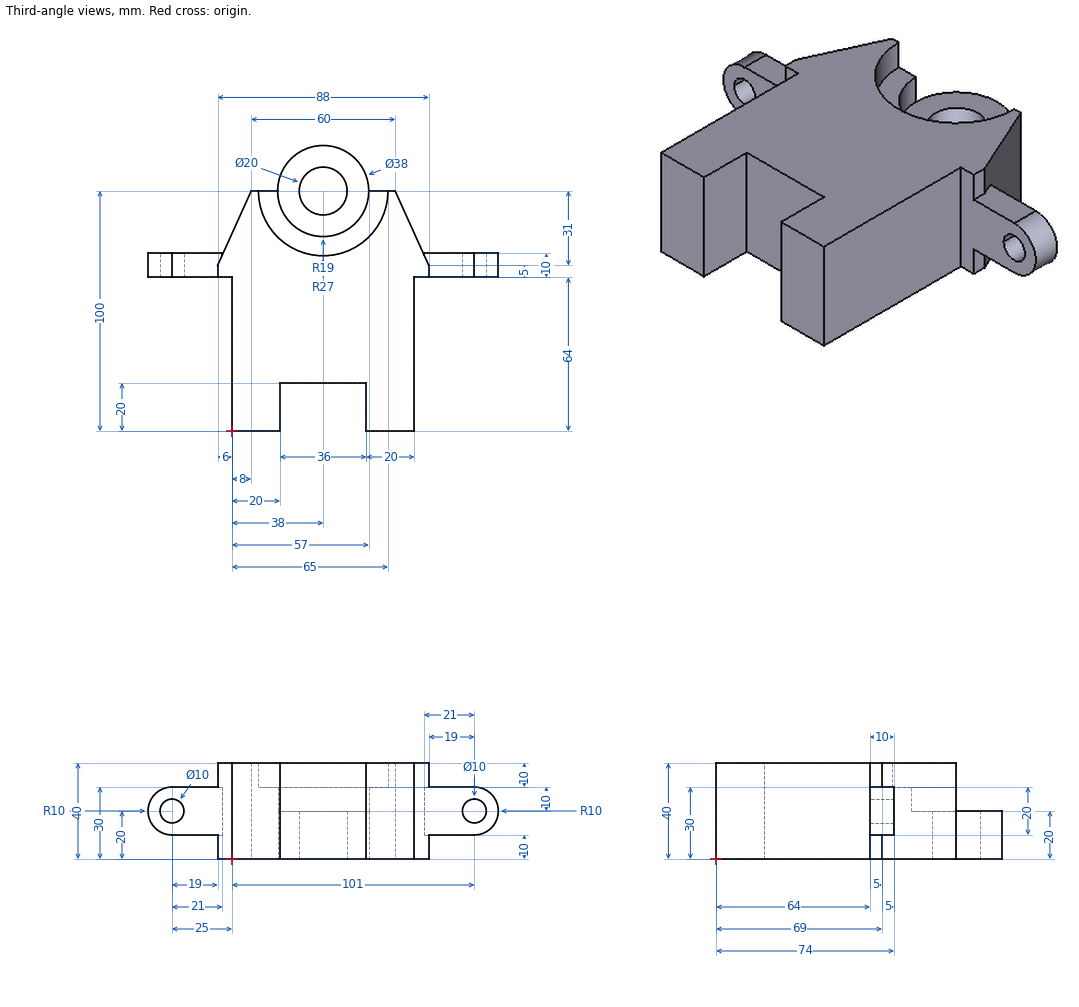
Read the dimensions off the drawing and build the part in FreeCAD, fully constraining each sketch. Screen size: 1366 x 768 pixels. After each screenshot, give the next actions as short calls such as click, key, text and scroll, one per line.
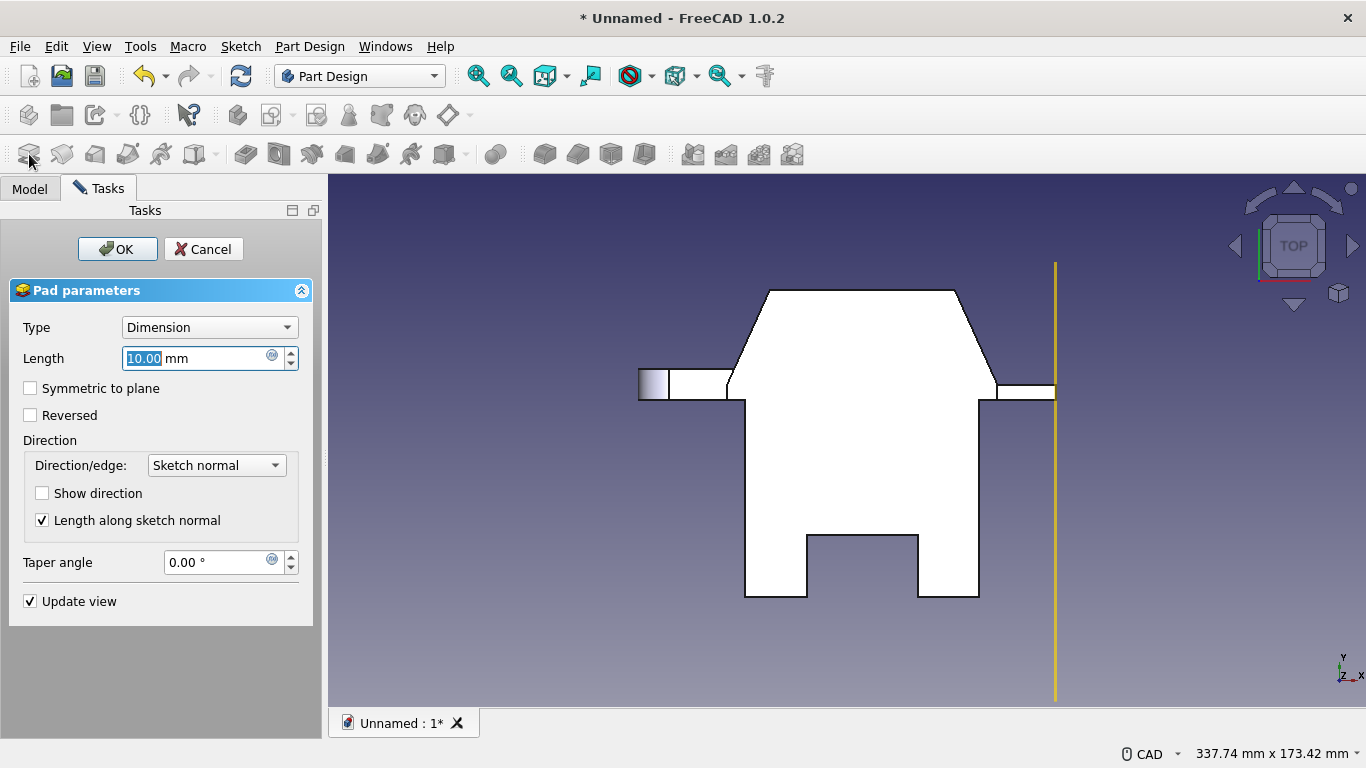
text(21)
key(Tab)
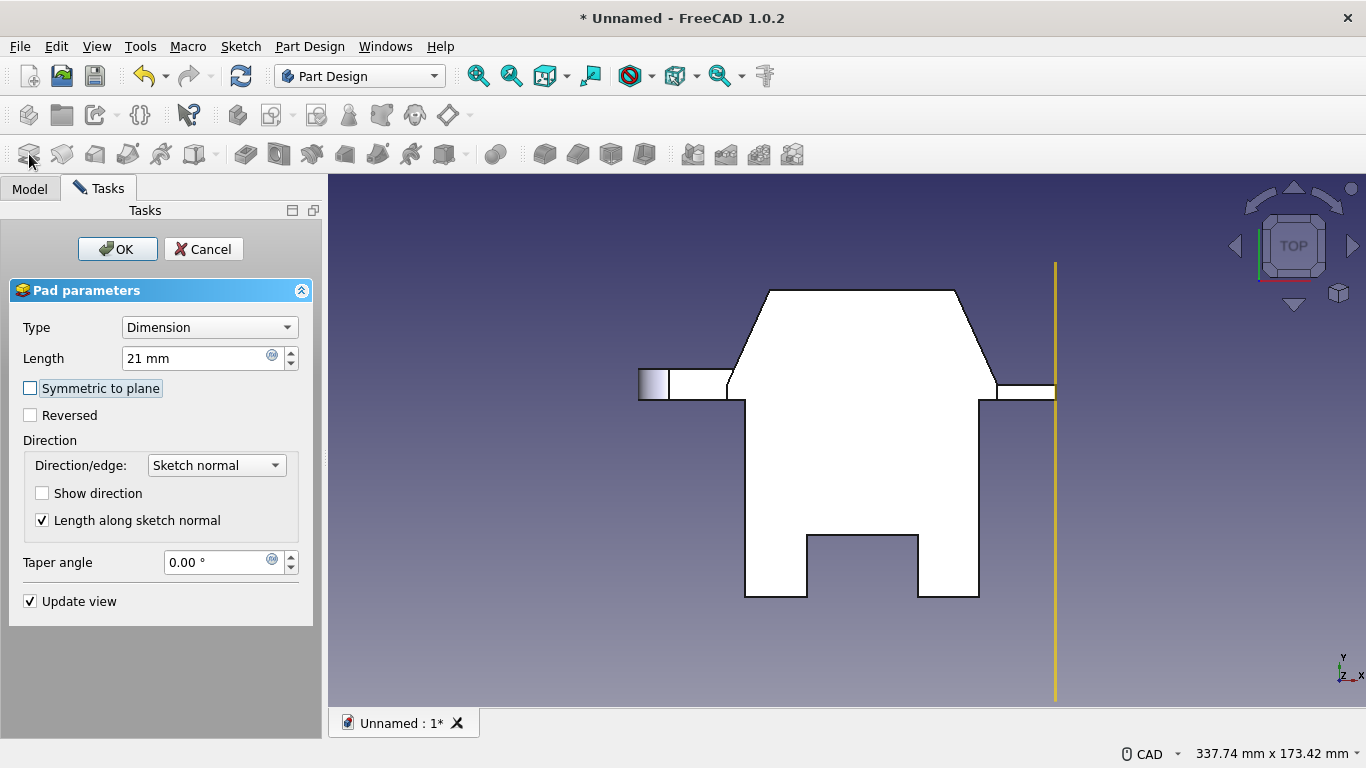
click(31, 415)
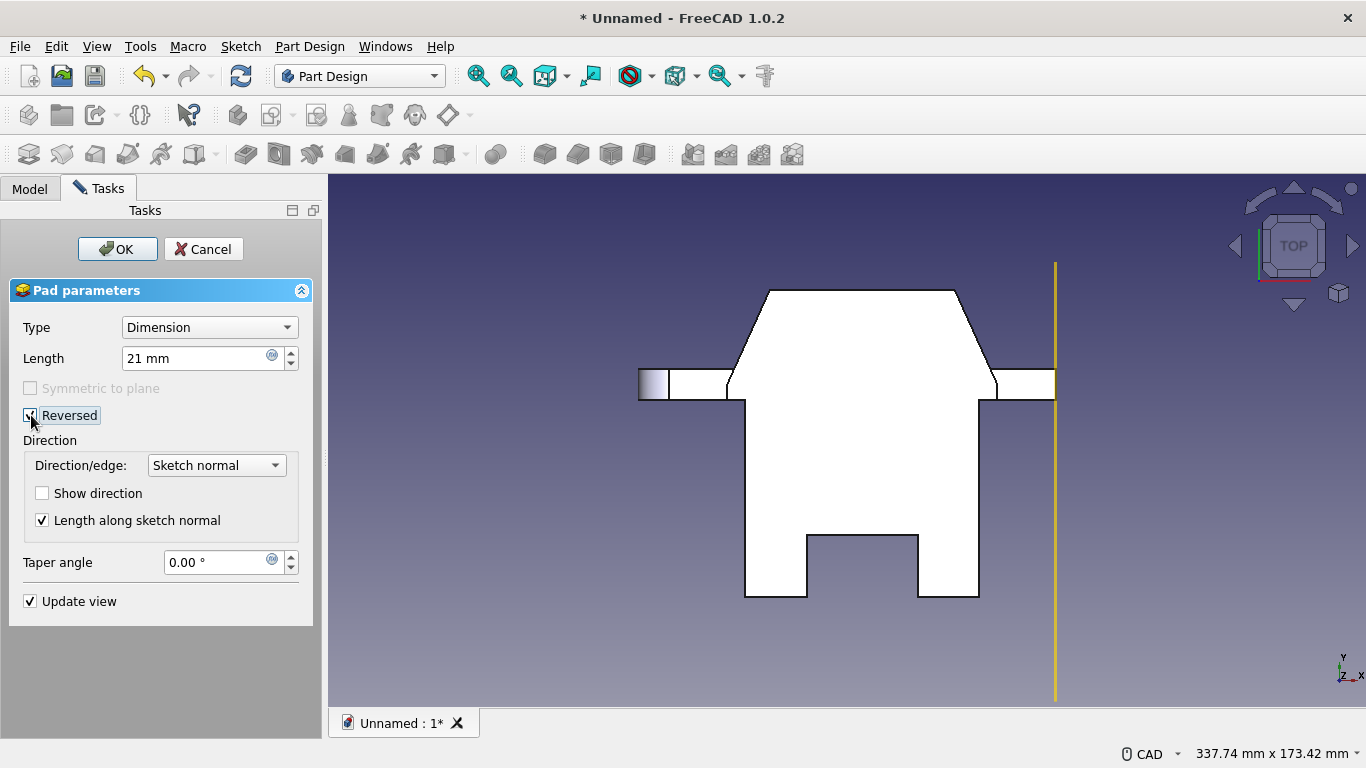
click(118, 249)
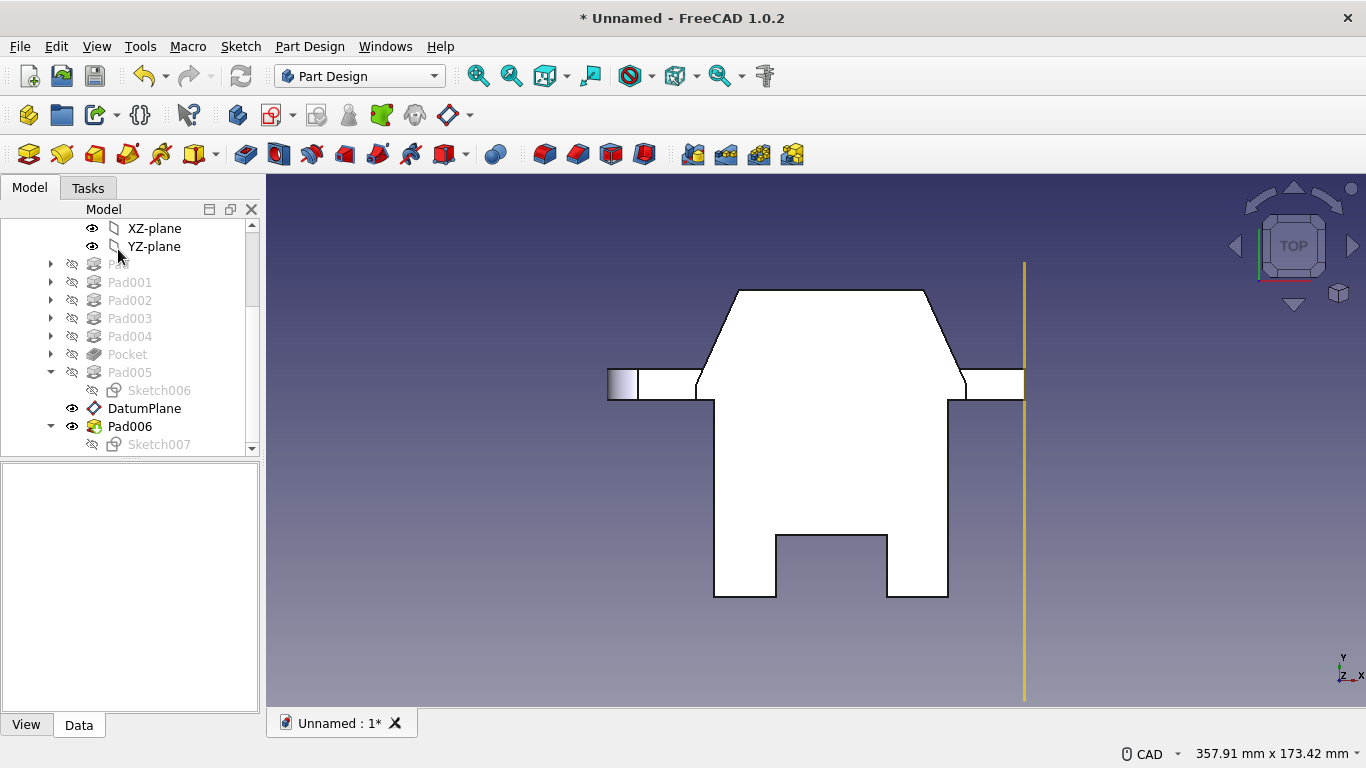
click(117, 408)
key(space)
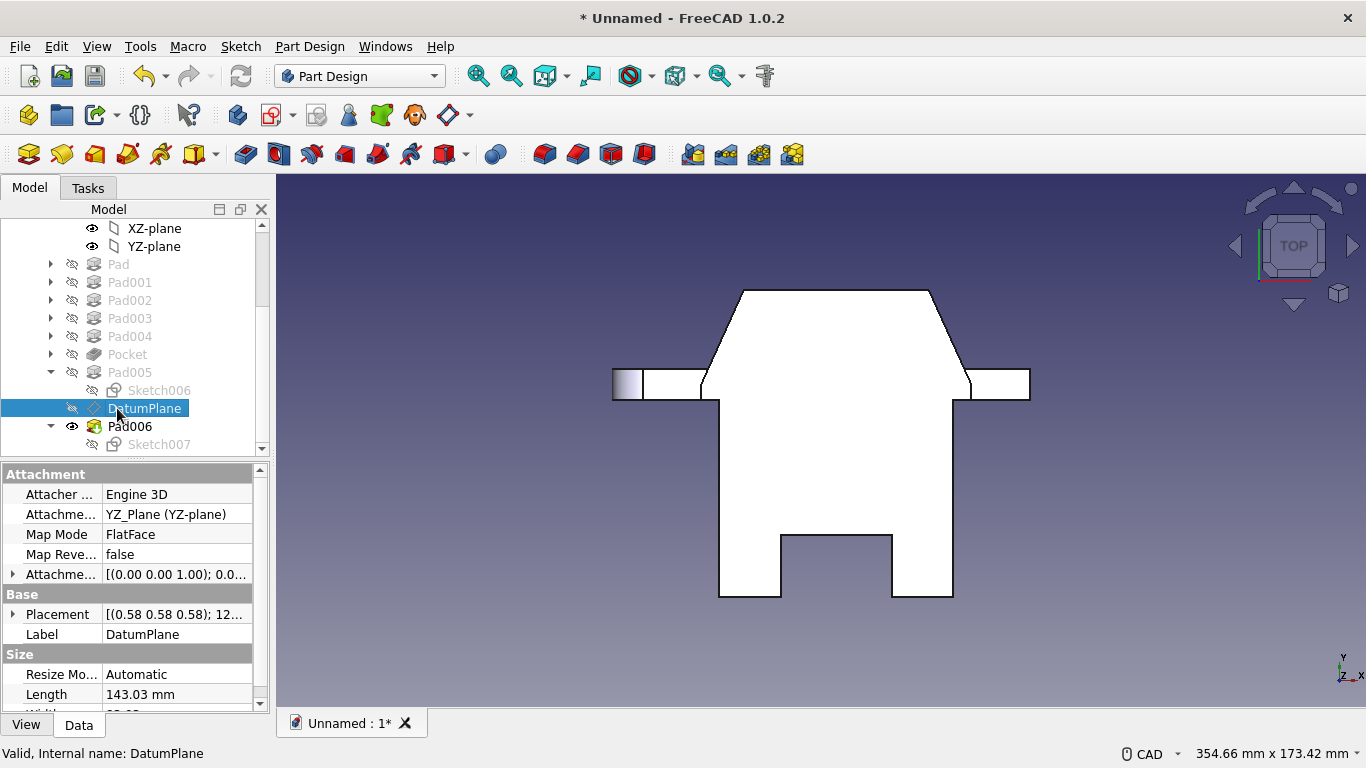
key(4)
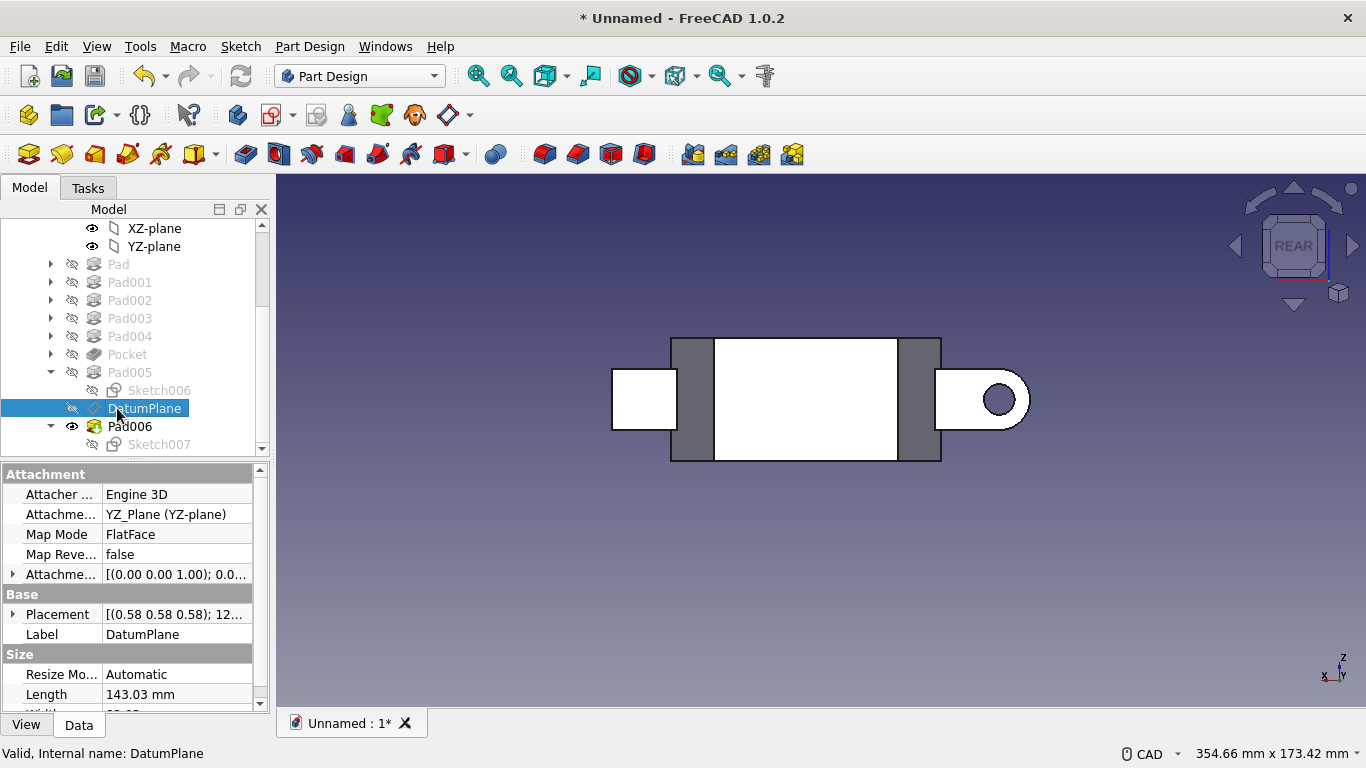
click(479, 76)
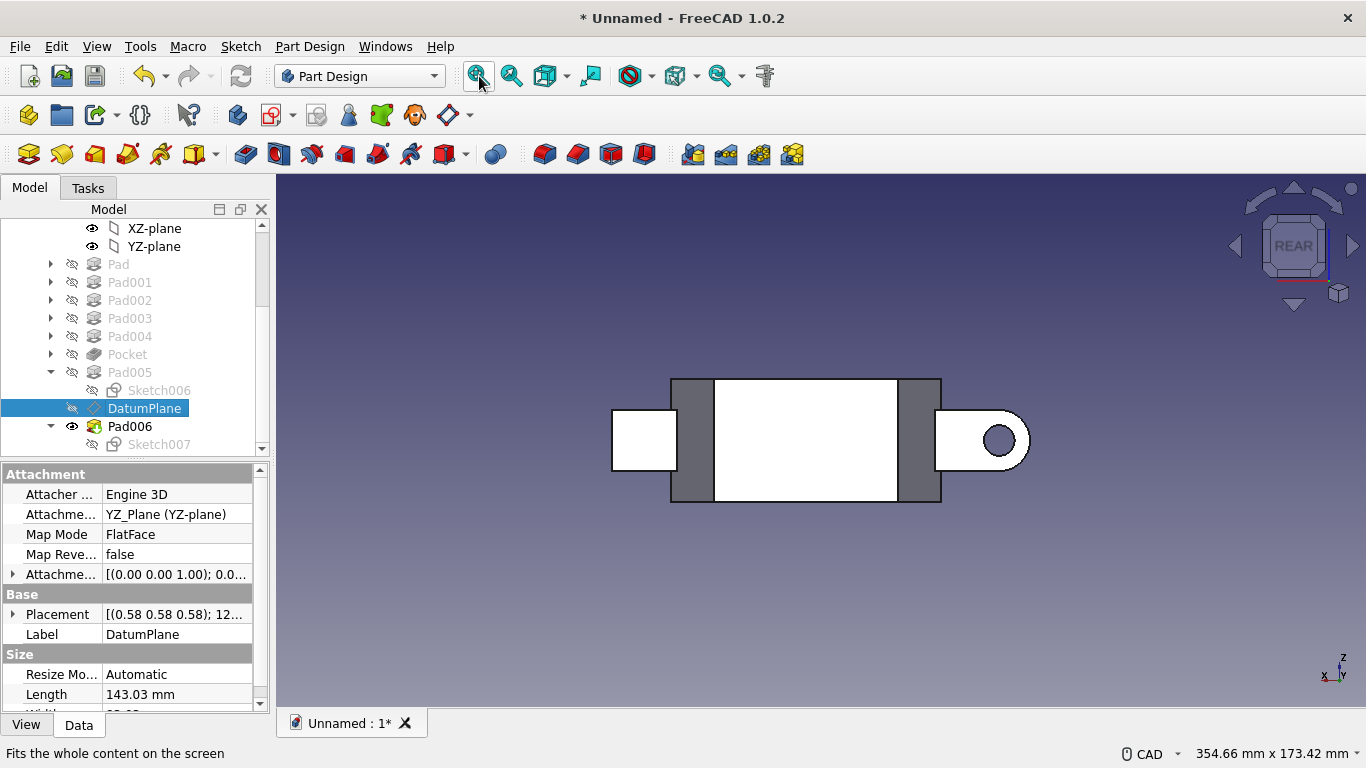
click(955, 431)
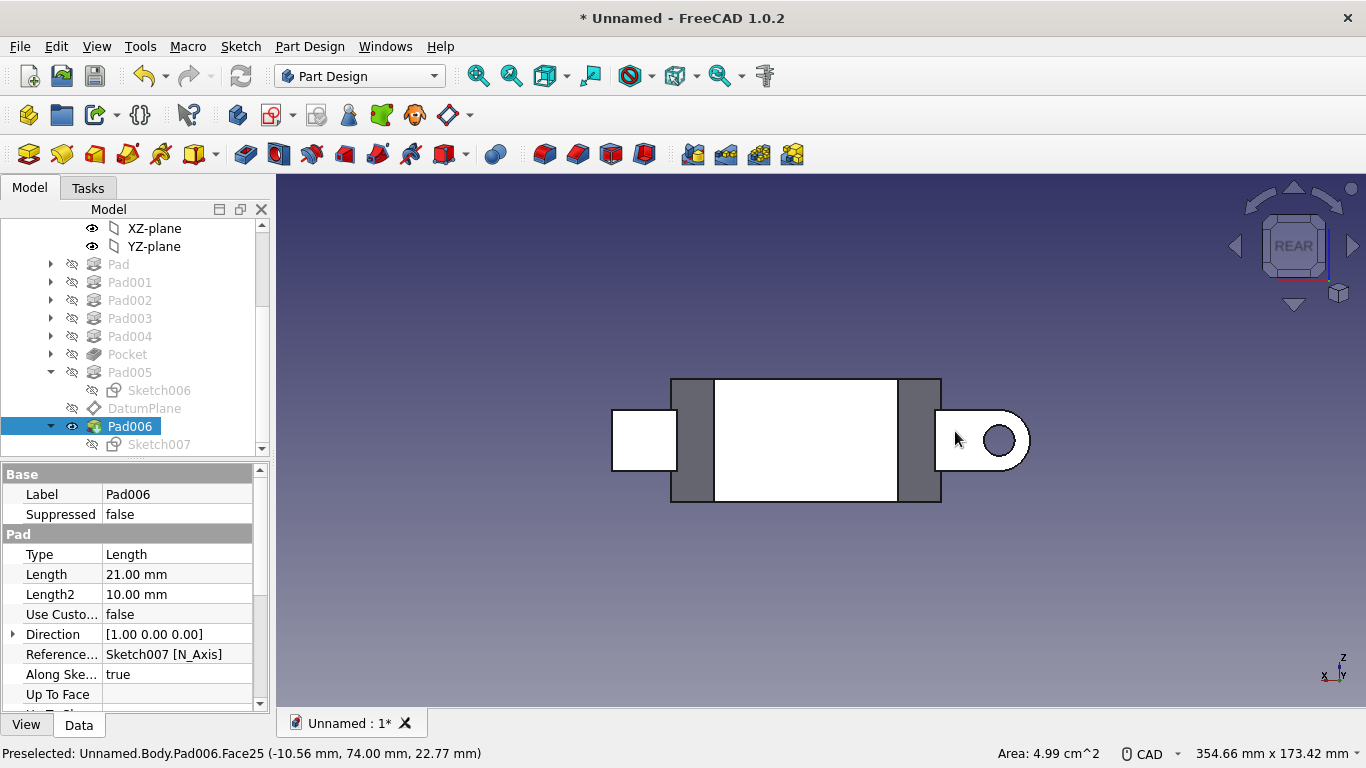
click(270, 116)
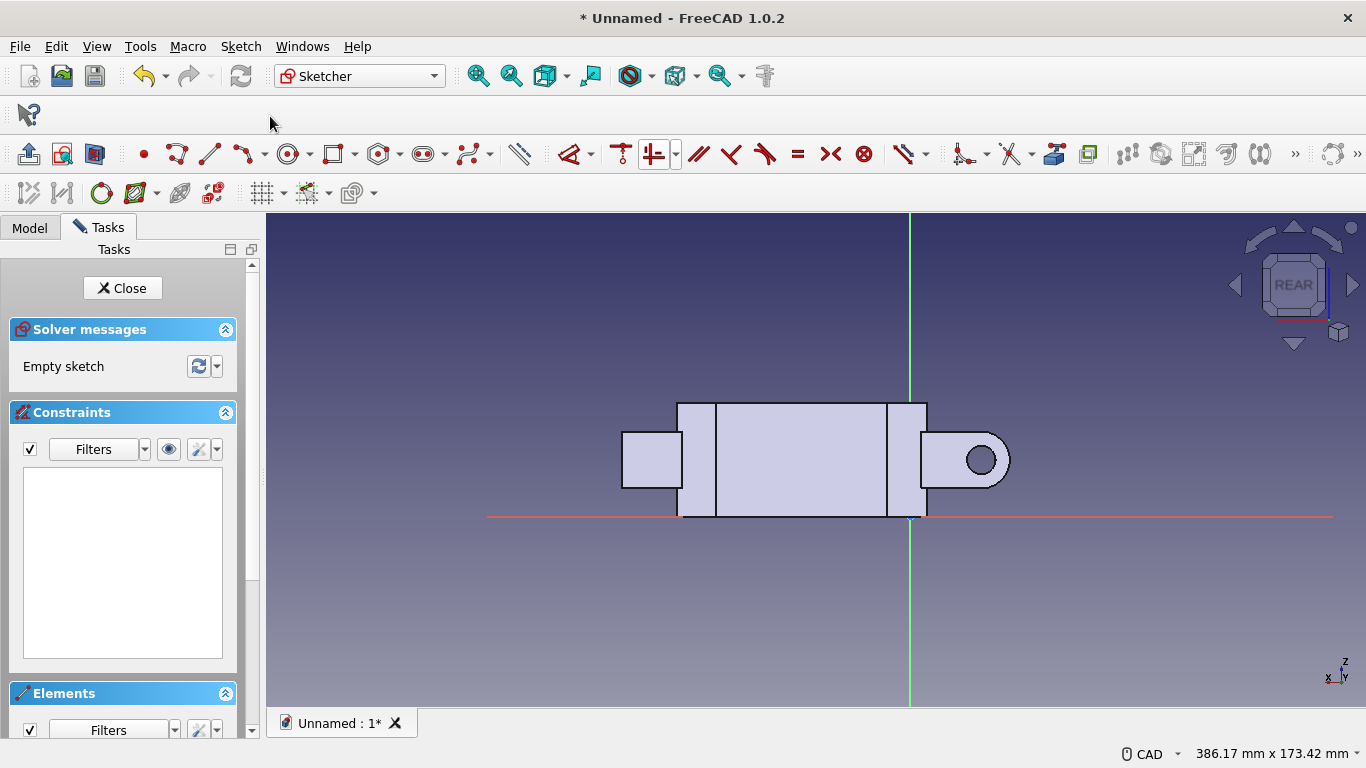
click(95, 154)